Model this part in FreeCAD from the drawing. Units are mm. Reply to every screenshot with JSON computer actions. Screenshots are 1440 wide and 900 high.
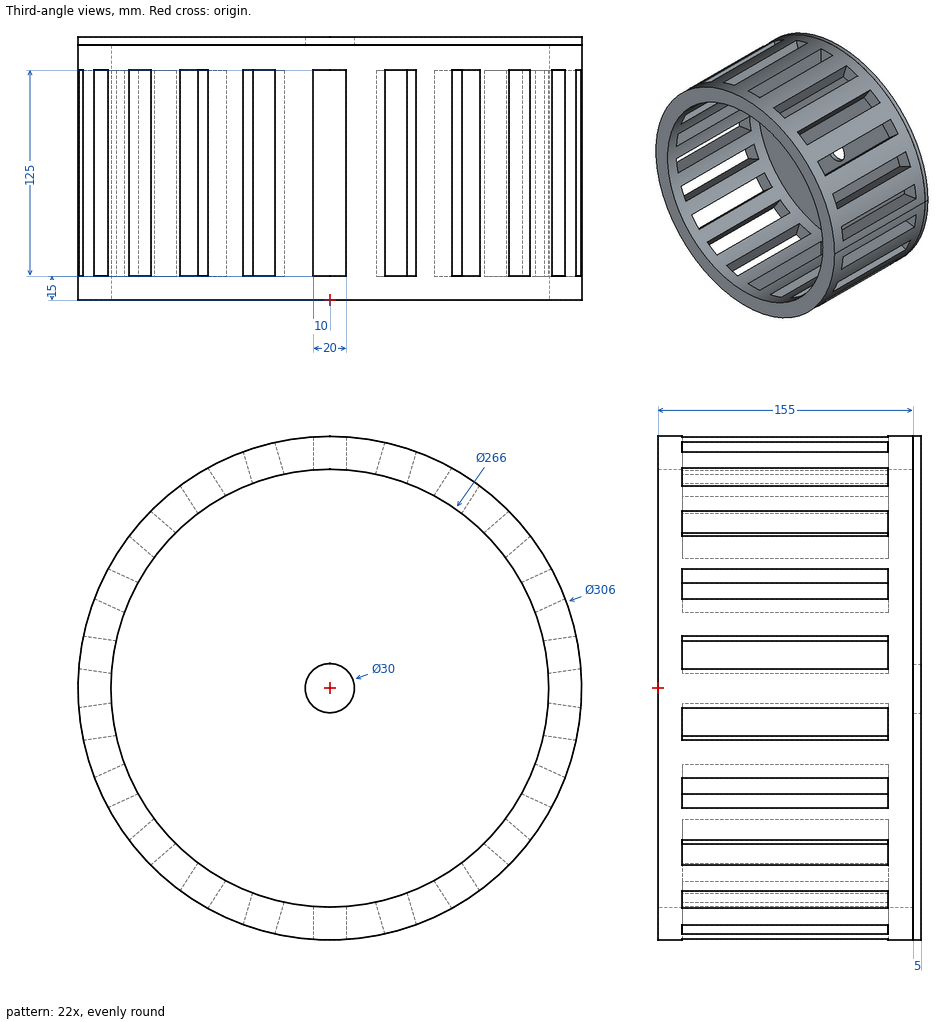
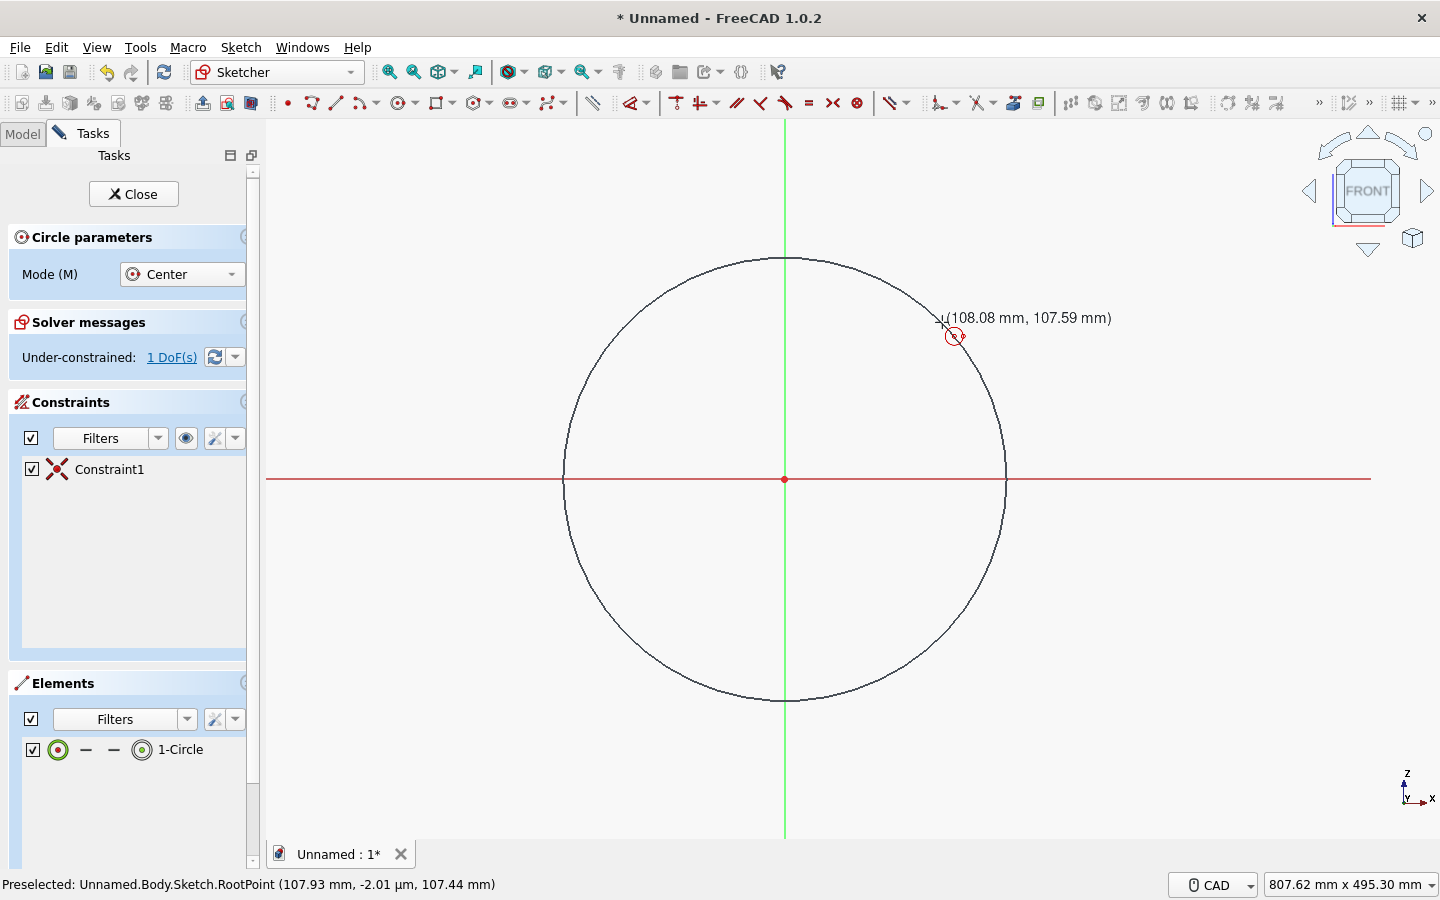
{"action": "left_click", "coordinate": [785, 479]}
{"action": "left_click", "coordinate": [922, 343]}
{"action": "key", "text": "Escape"}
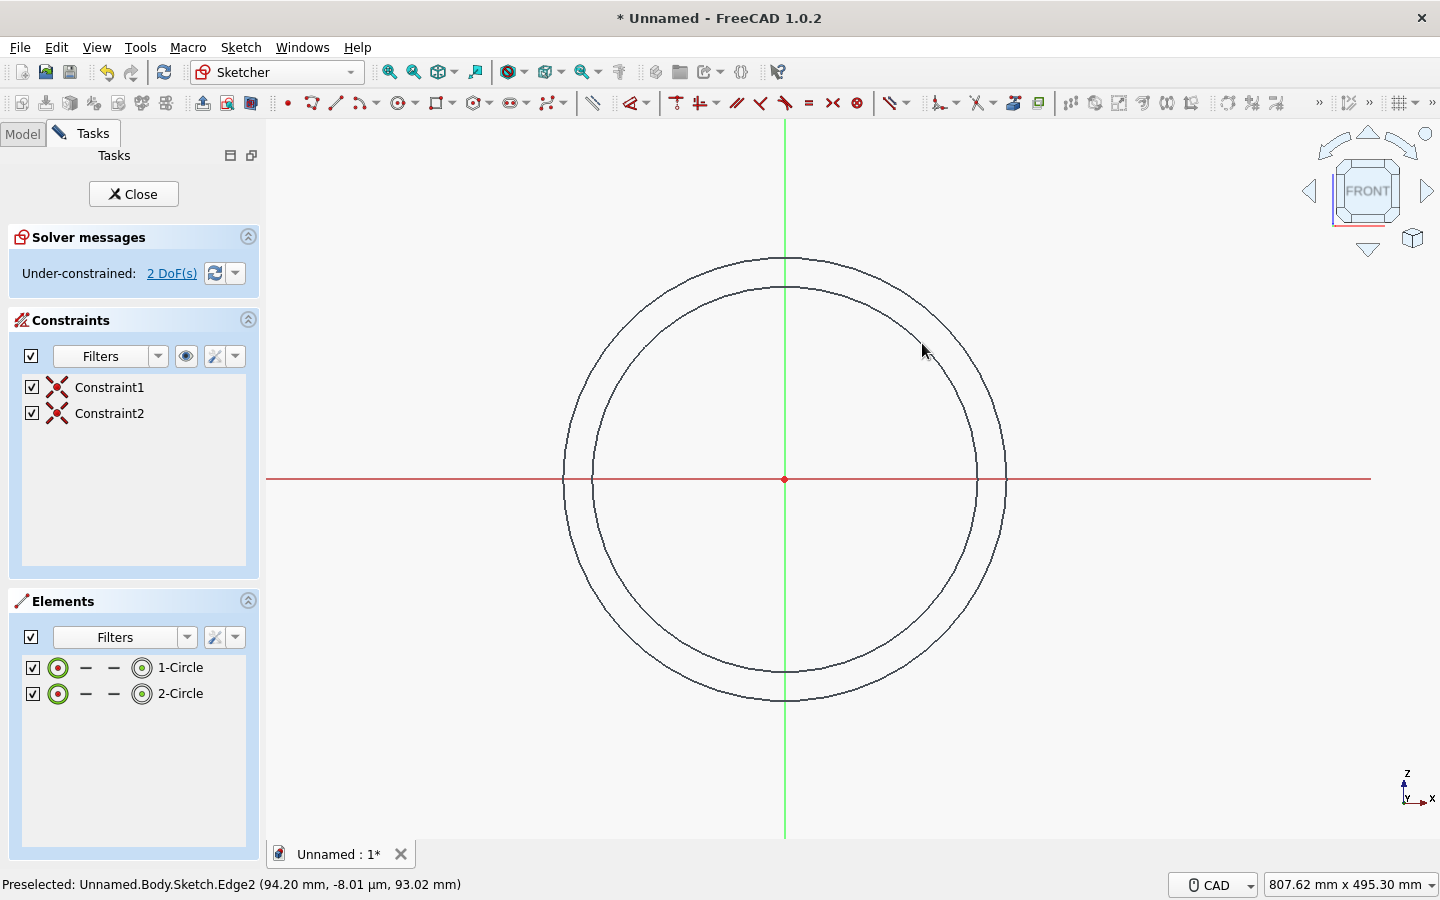
{"action": "left_click", "coordinate": [630, 104]}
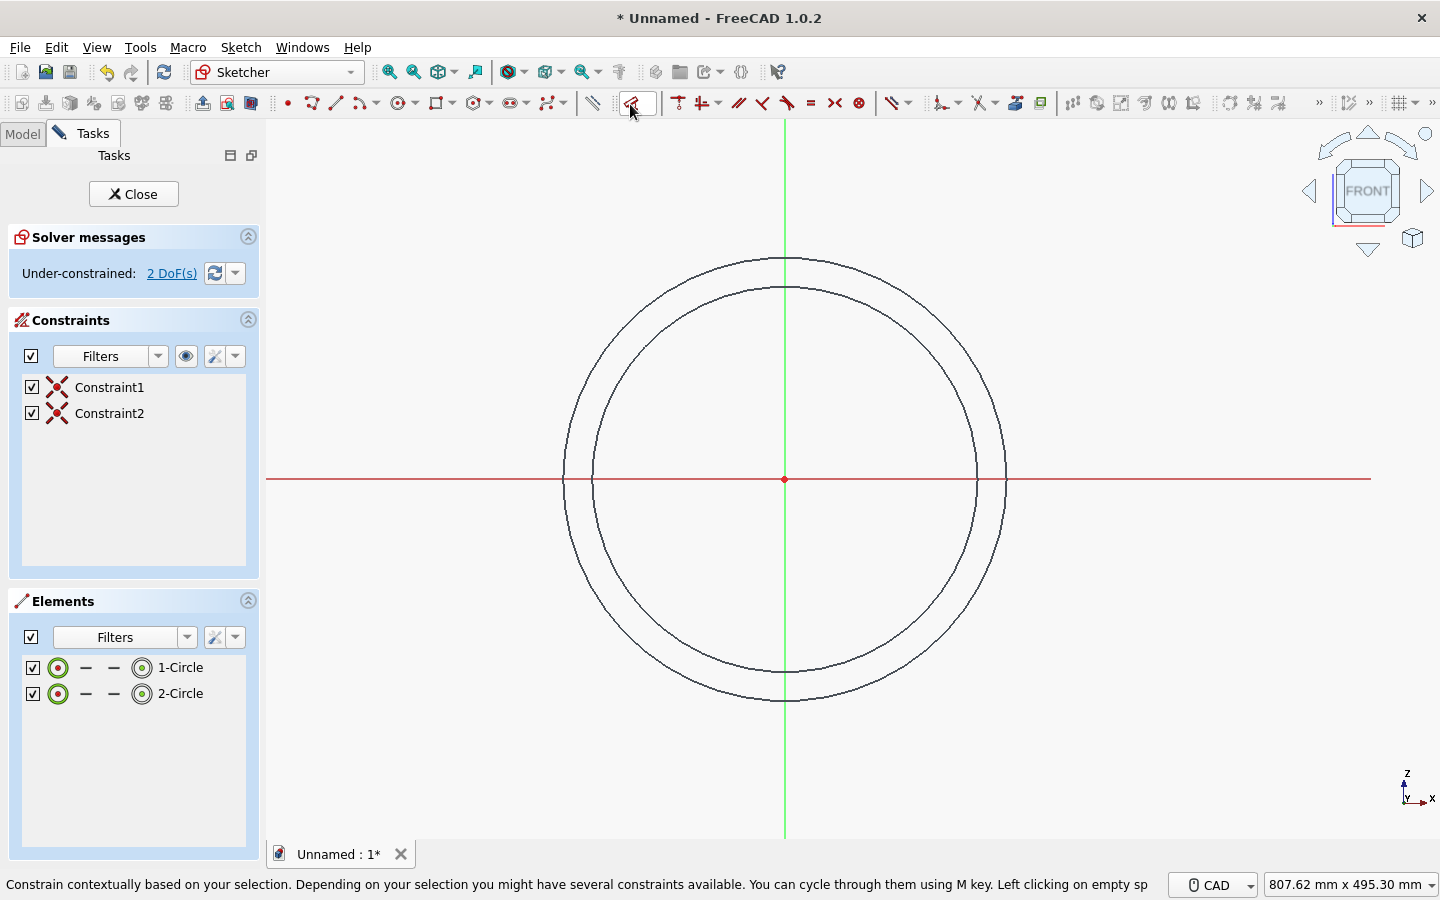
{"action": "left_click", "coordinate": [941, 322]}
{"action": "left_click", "coordinate": [964, 299]}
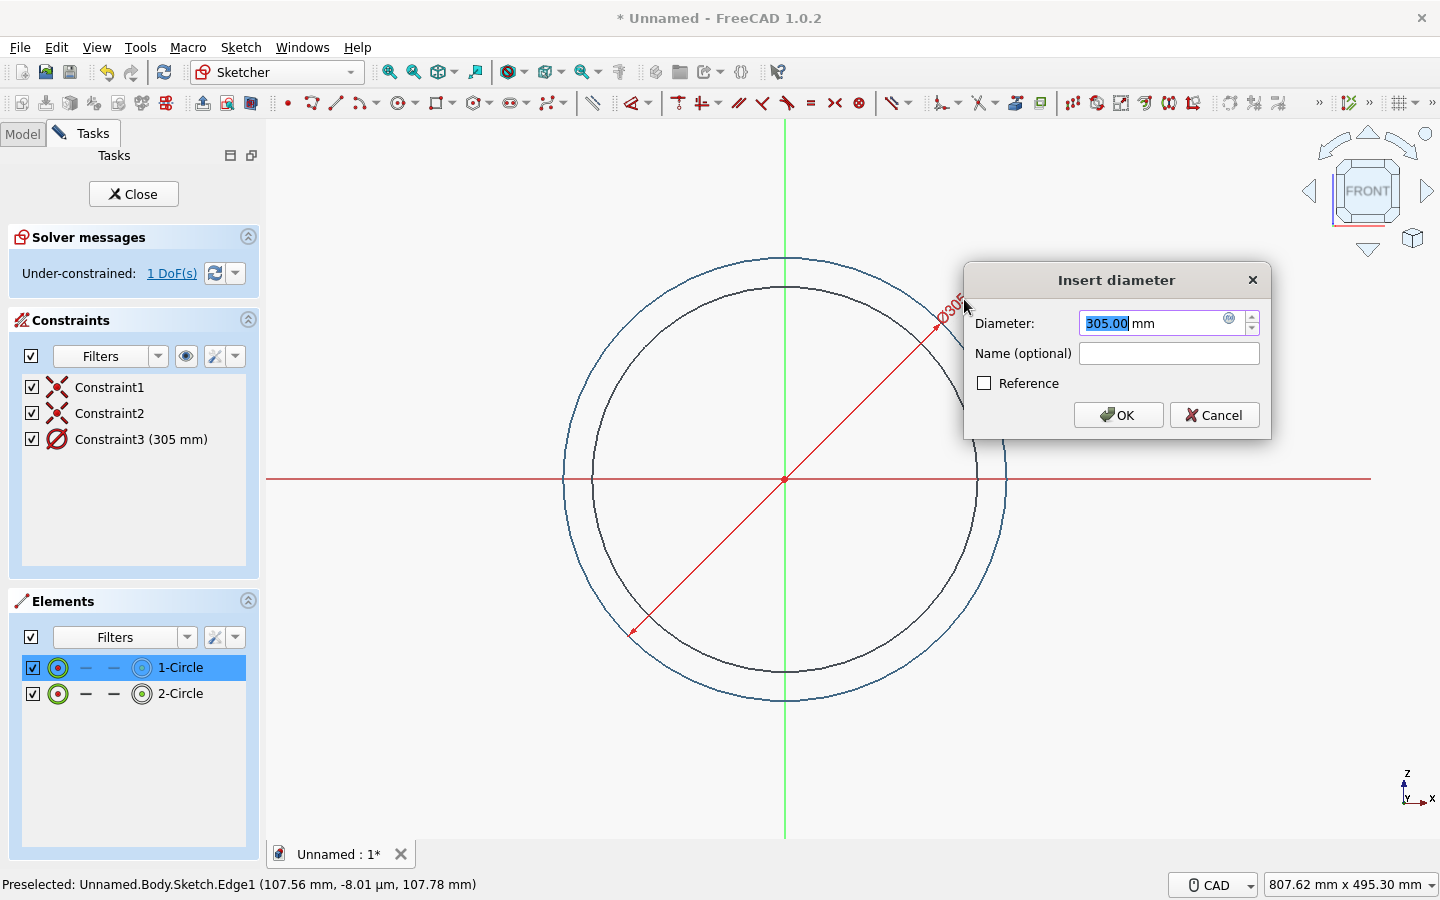
{"action": "type", "text": "306"}
{"action": "key", "text": "Return"}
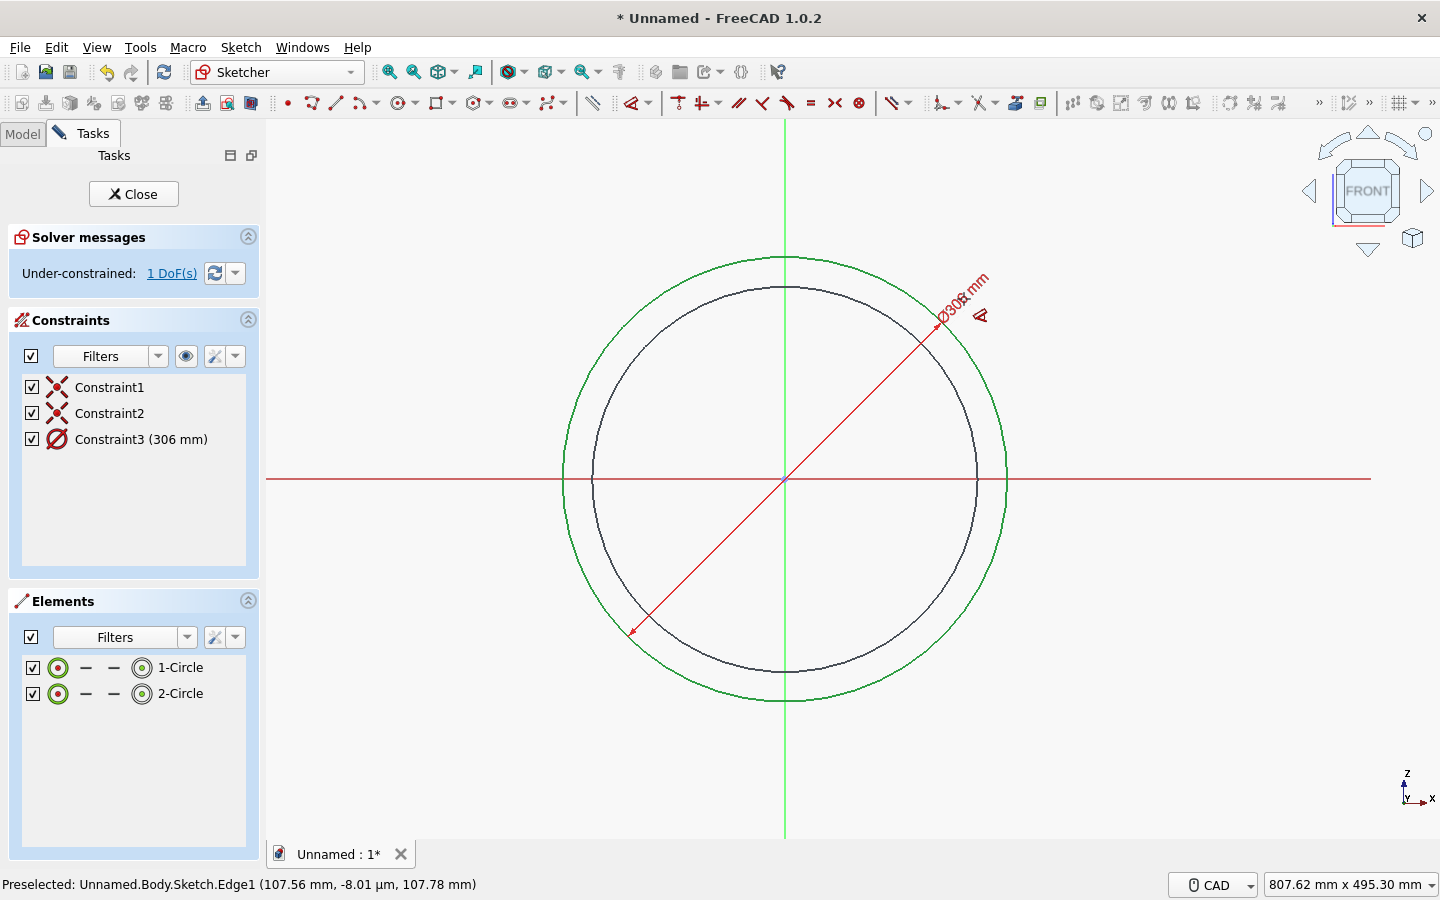
{"action": "left_click", "coordinate": [921, 343]}
{"action": "left_click", "coordinate": [1022, 409]}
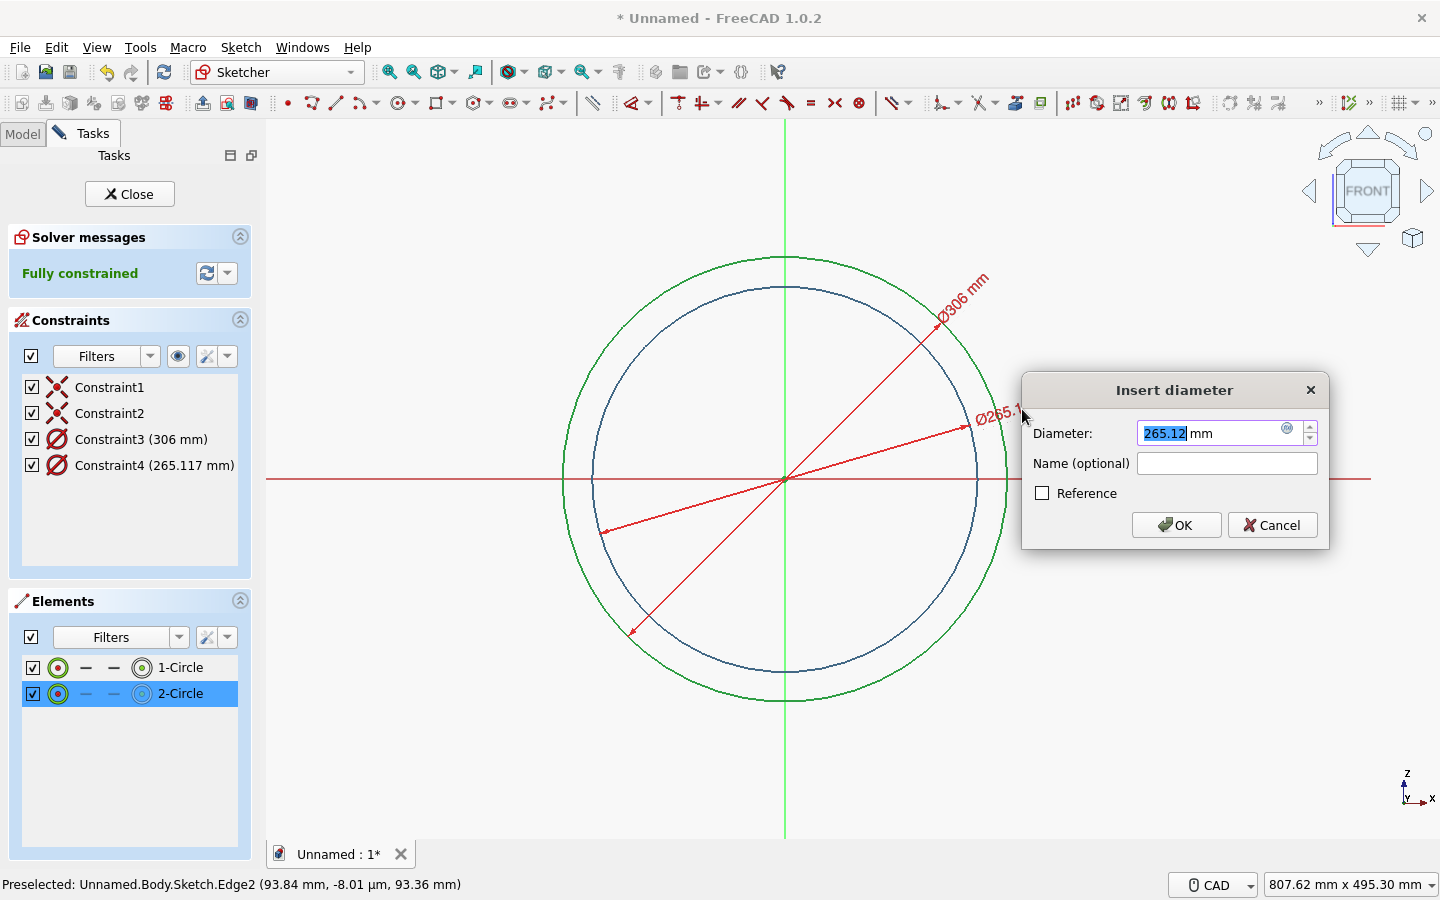
{"action": "type", "text": "266"}
{"action": "key", "text": "Return"}
{"action": "key", "text": "Escape"}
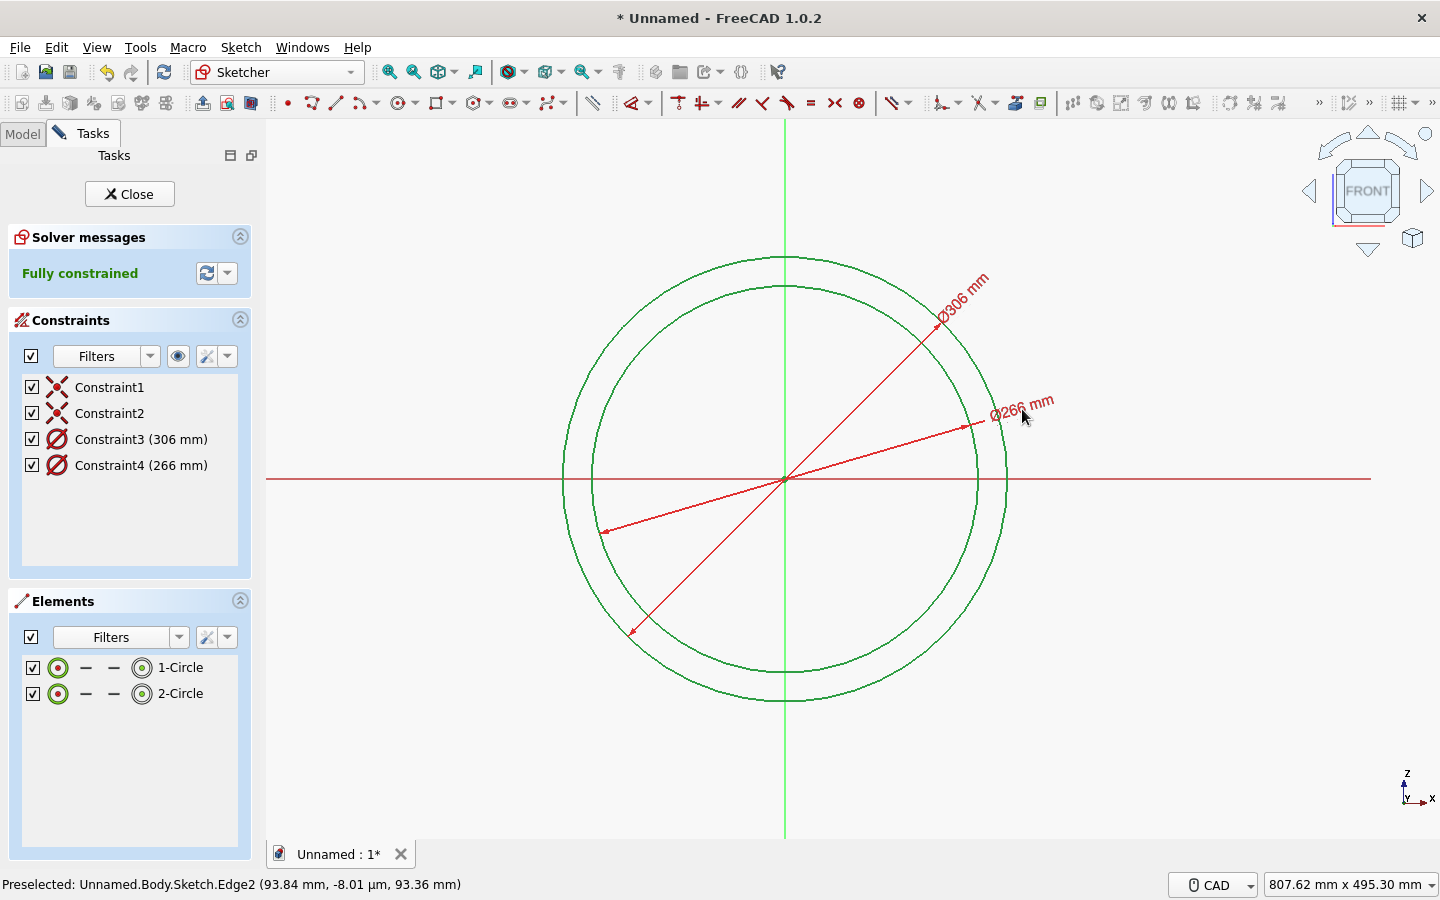
{"action": "left_click", "coordinate": [130, 194]}